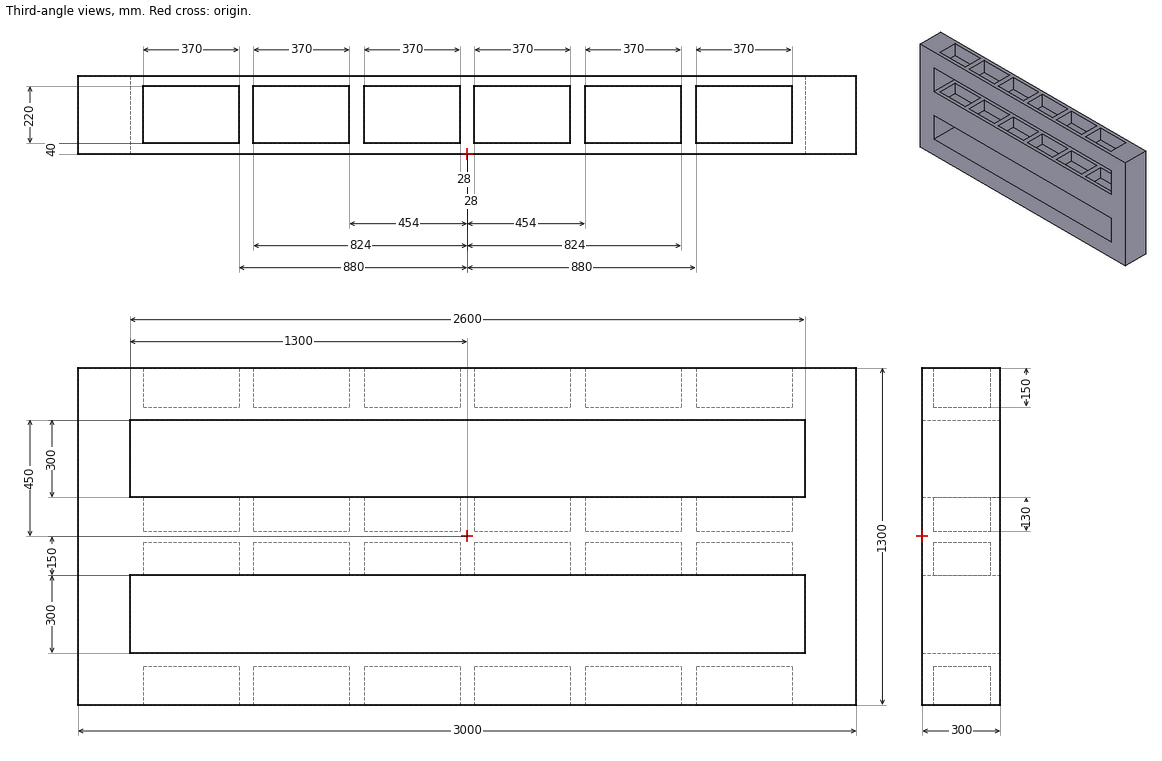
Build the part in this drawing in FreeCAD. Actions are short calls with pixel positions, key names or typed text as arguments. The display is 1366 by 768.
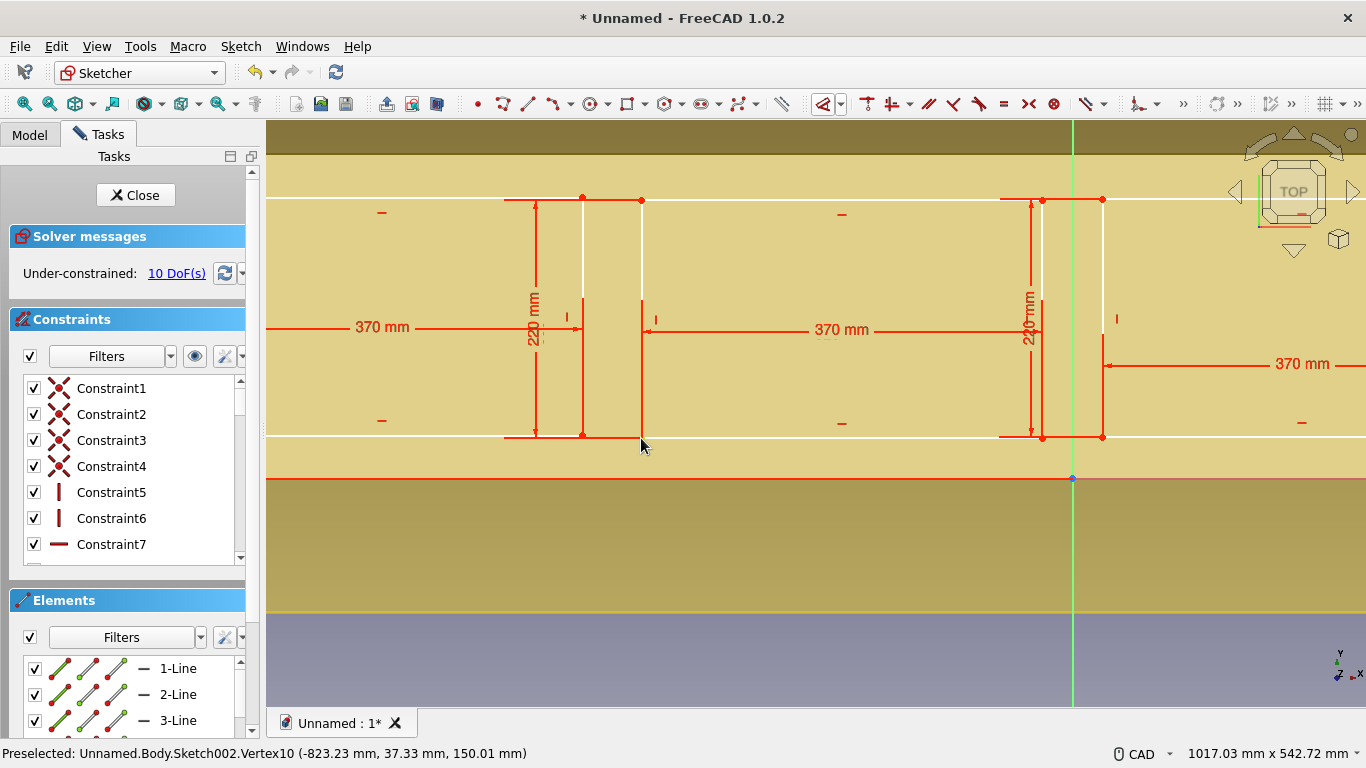
click(642, 438)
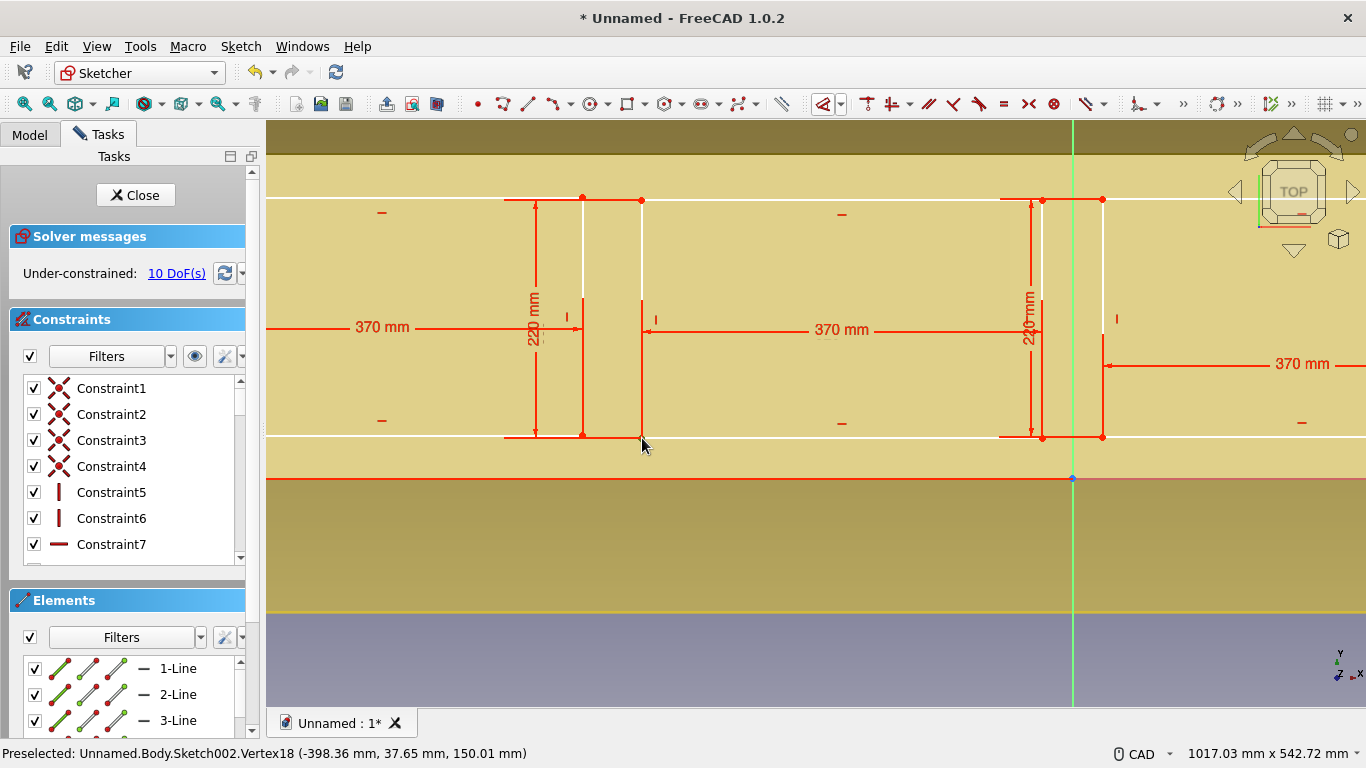
key(i)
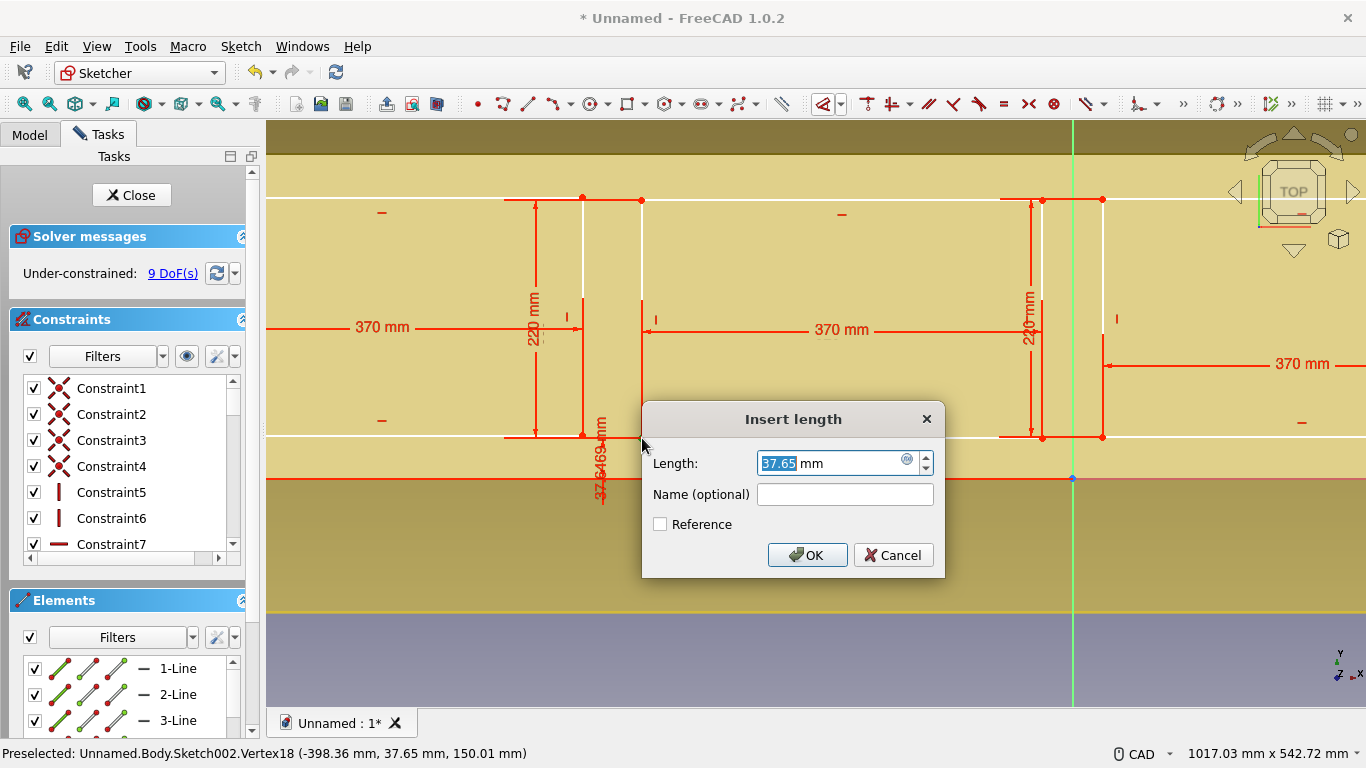
text(40)
key(Return)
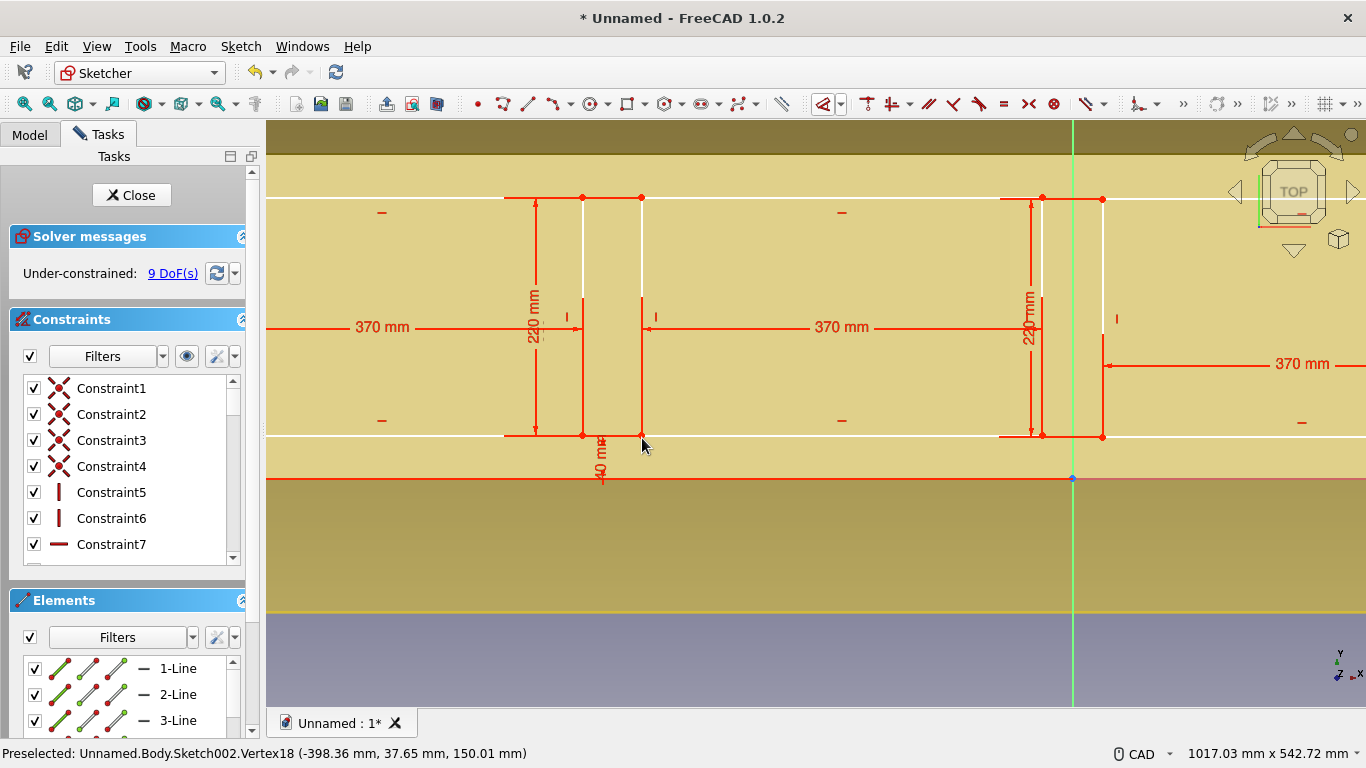
scroll(1042, 436, up, 2)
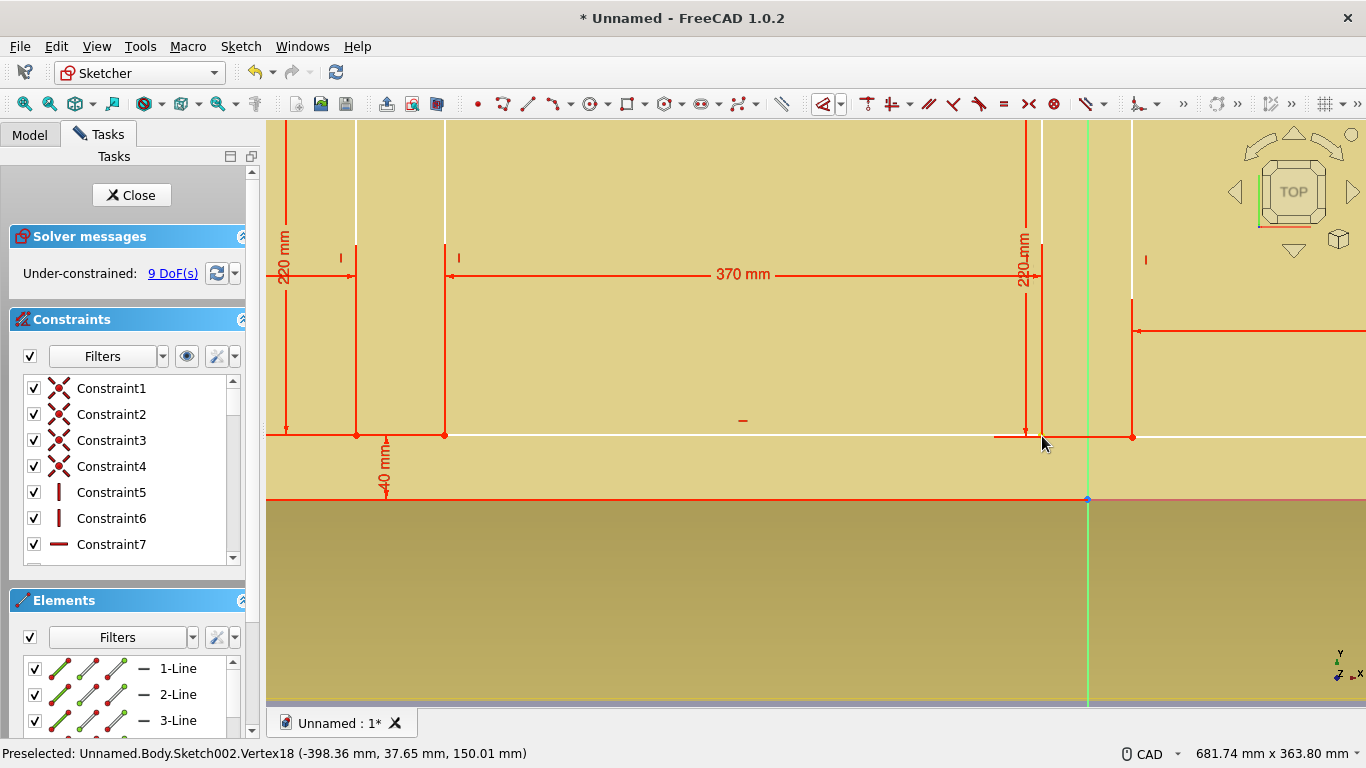
click(1042, 435)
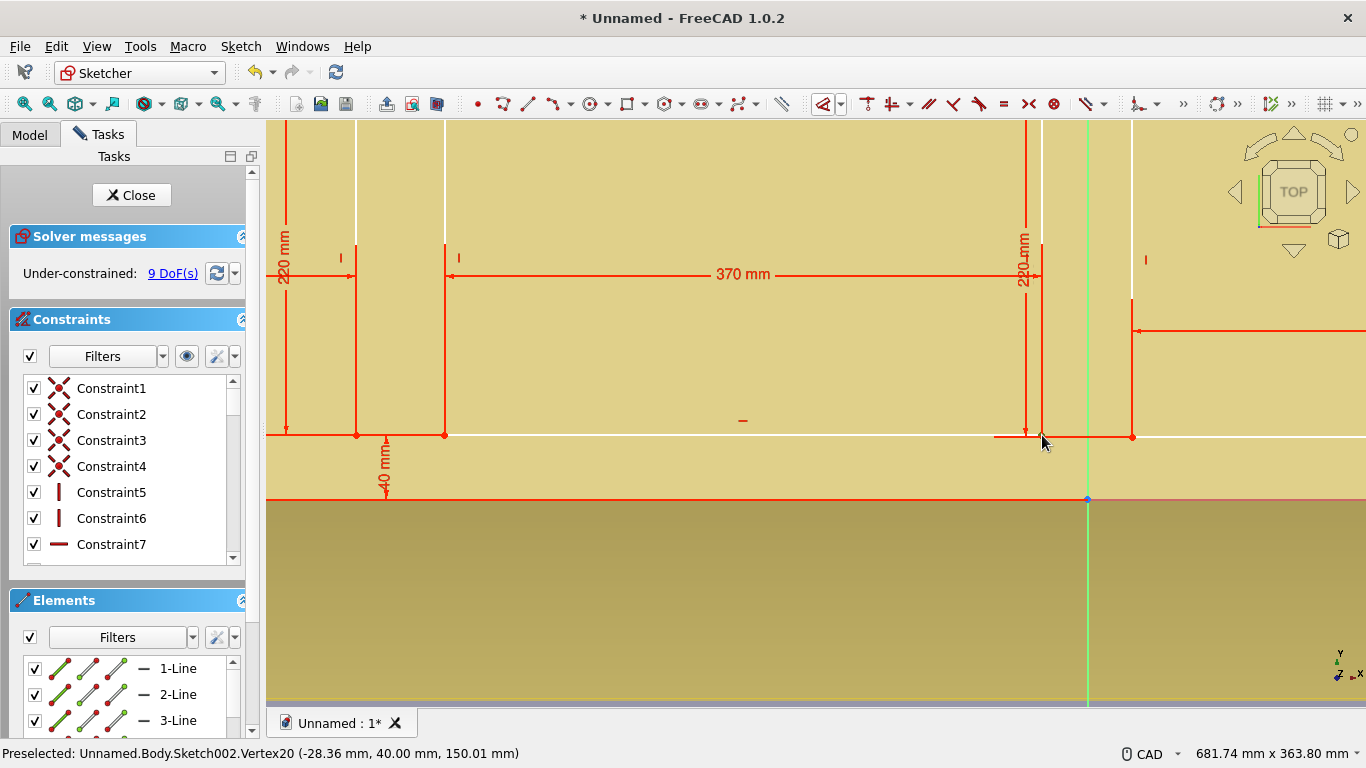
key(l)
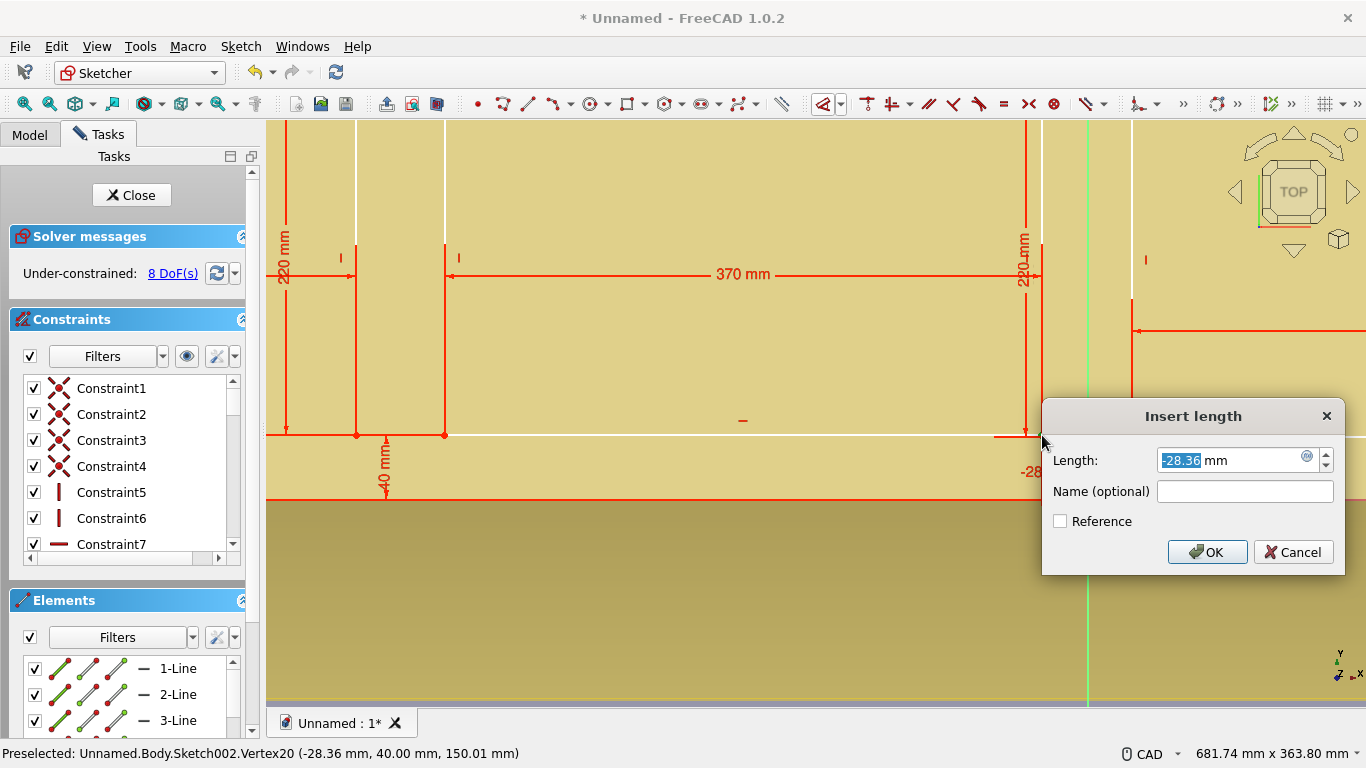
text(-28)
key(Return)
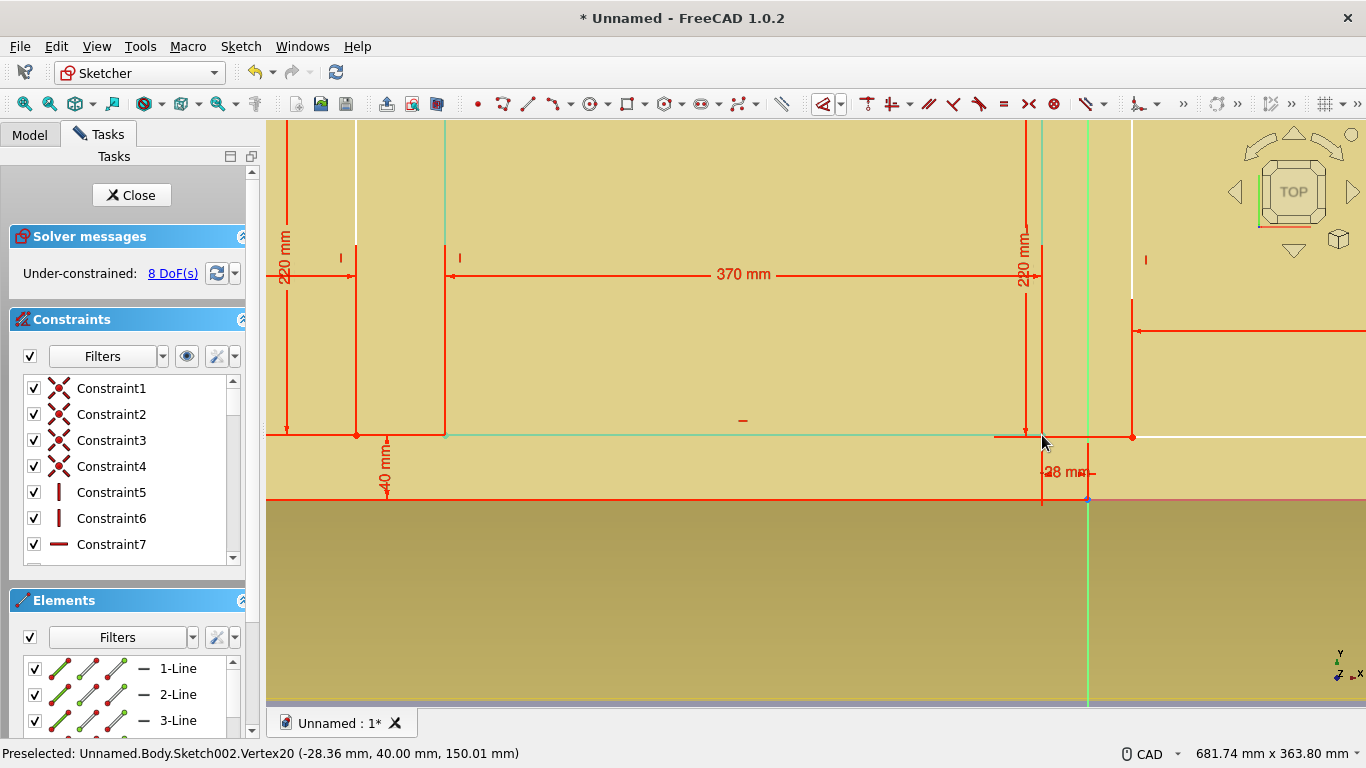
scroll(680, 438, down, 9)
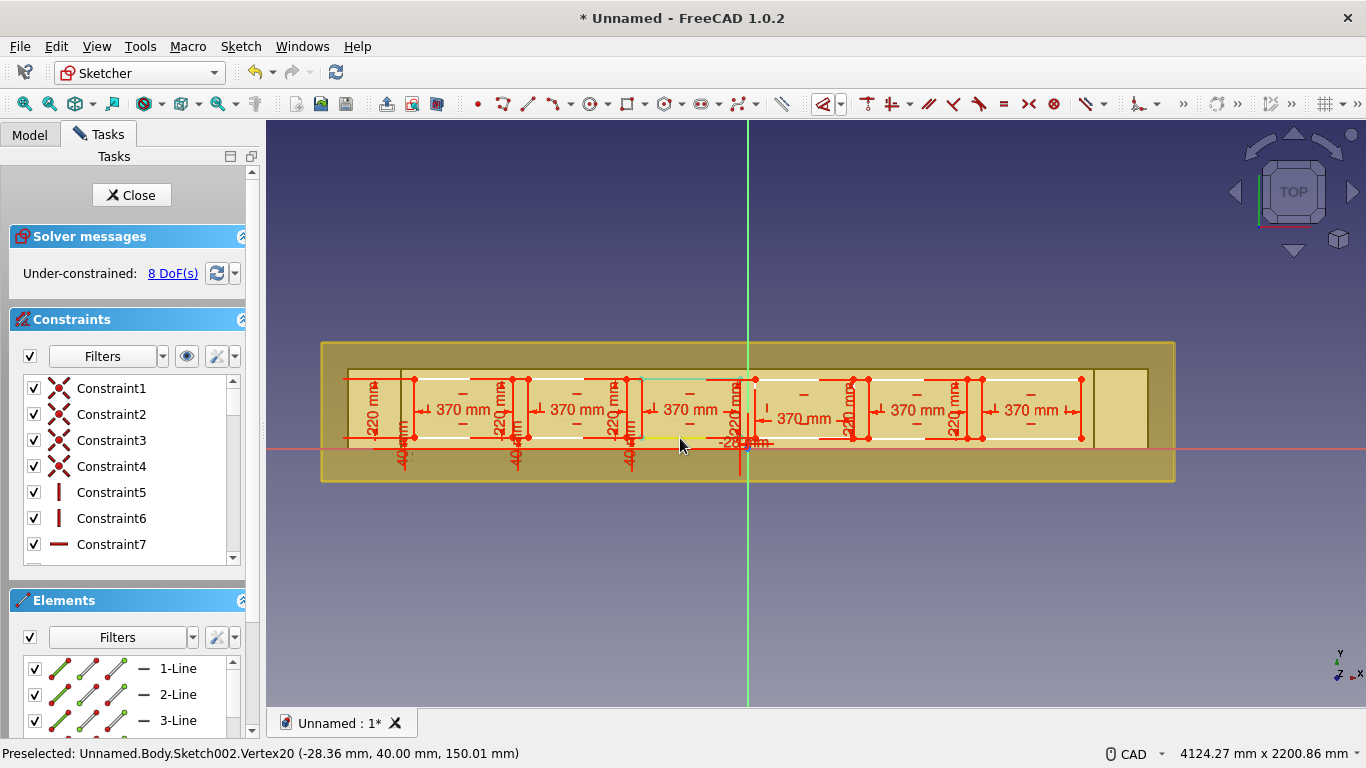
scroll(755, 380, up, 9)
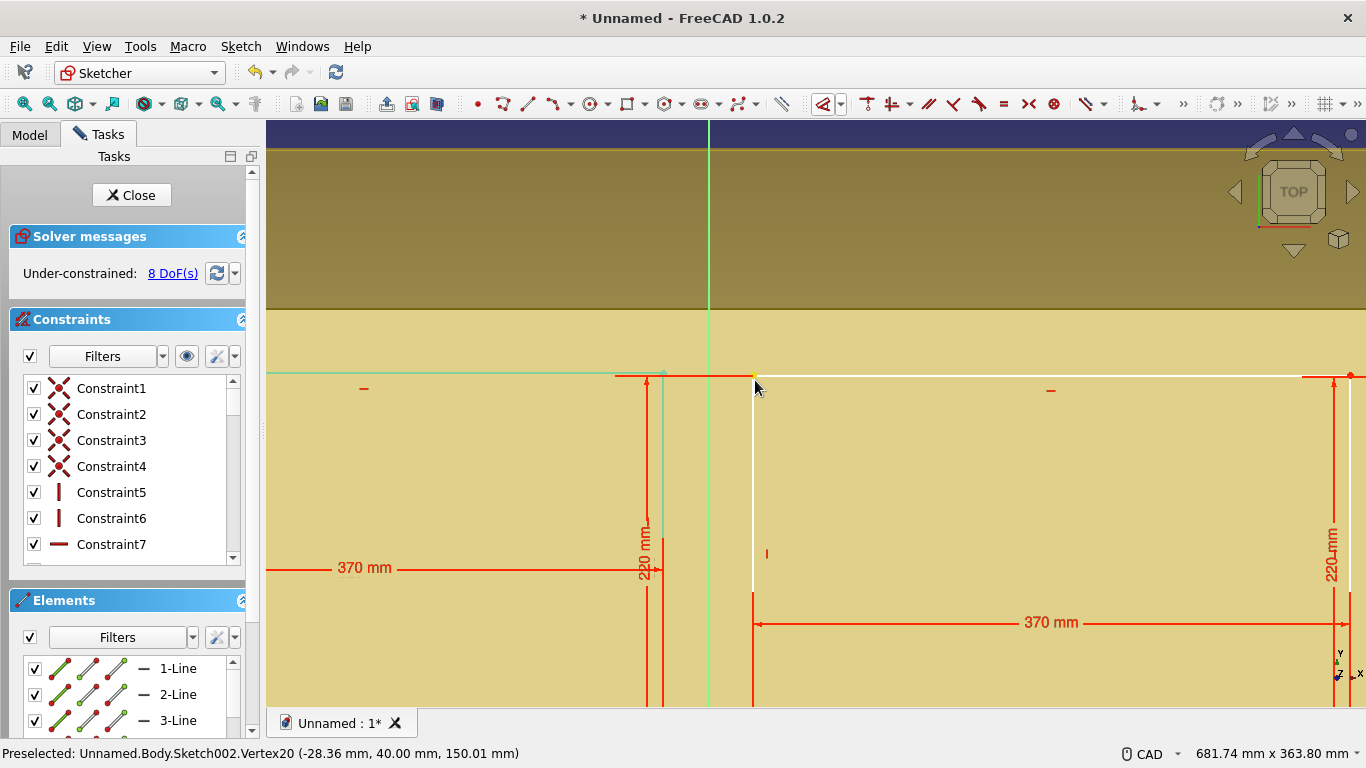
click(753, 376)